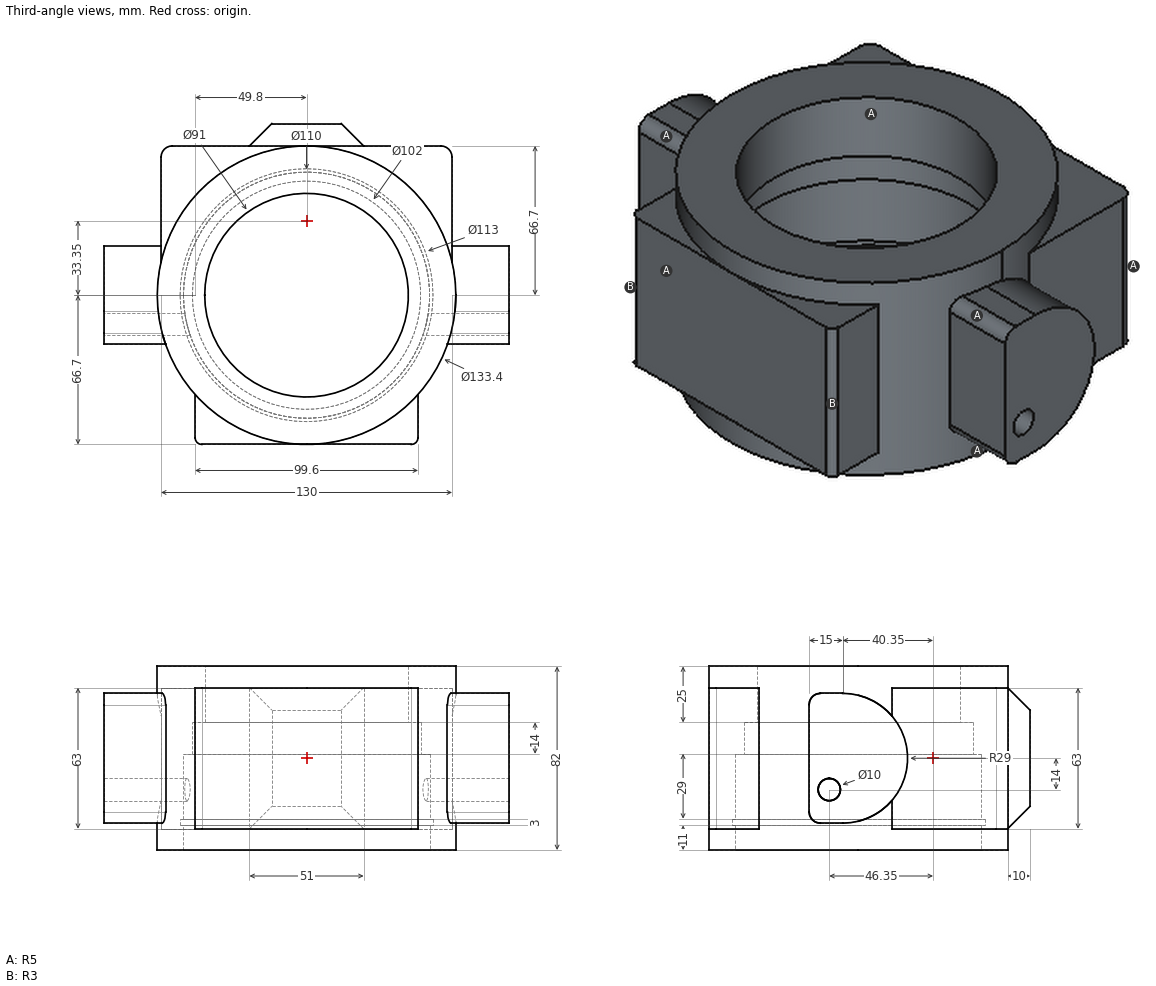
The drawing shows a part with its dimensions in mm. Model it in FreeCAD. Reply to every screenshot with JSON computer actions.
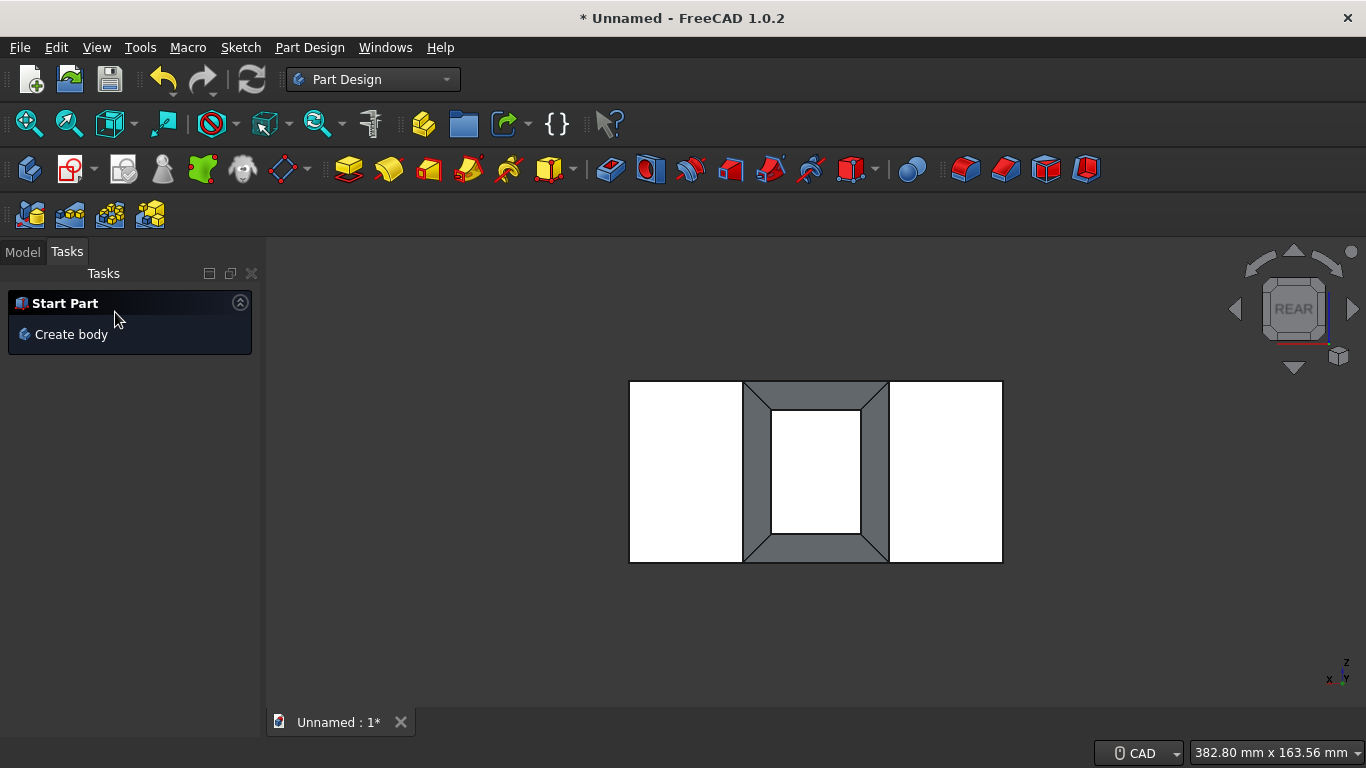
{"action": "left_click", "coordinate": [70, 170]}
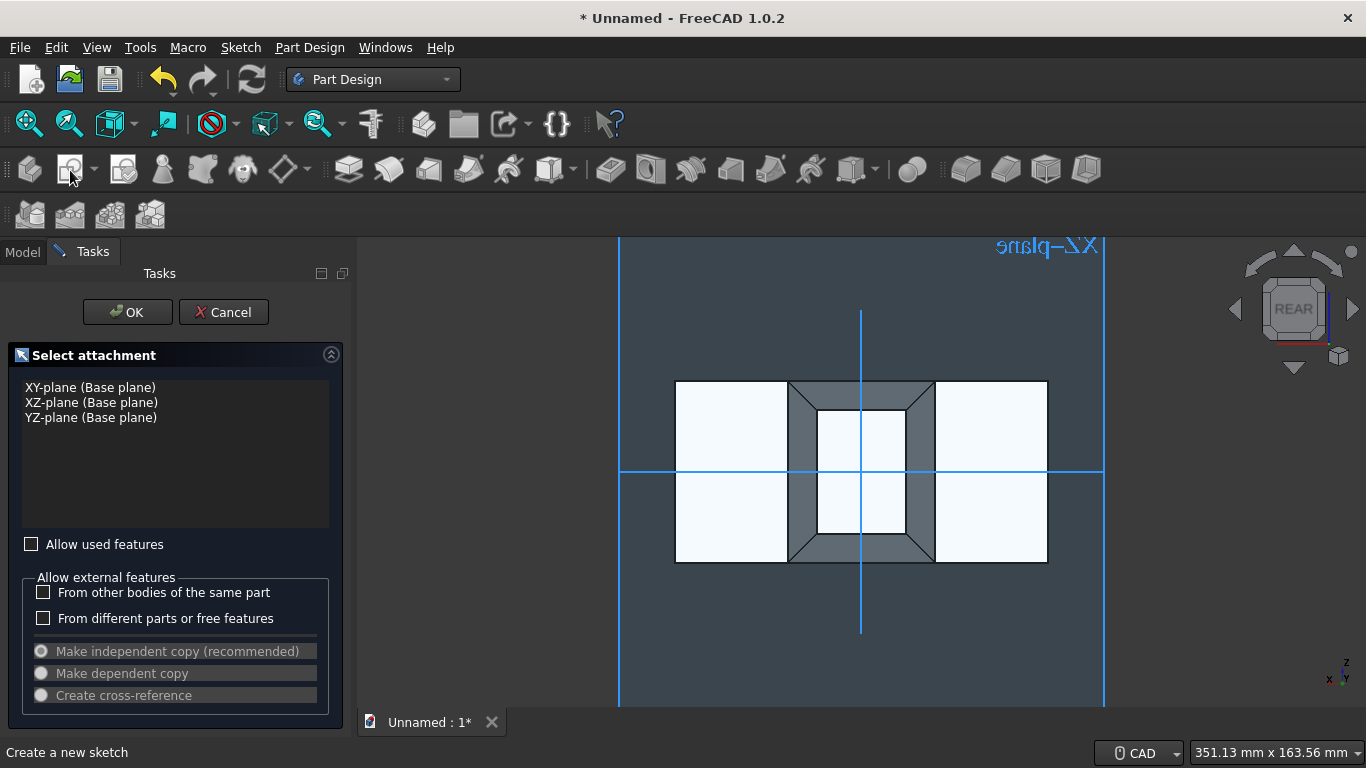
{"action": "left_click", "coordinate": [82, 388]}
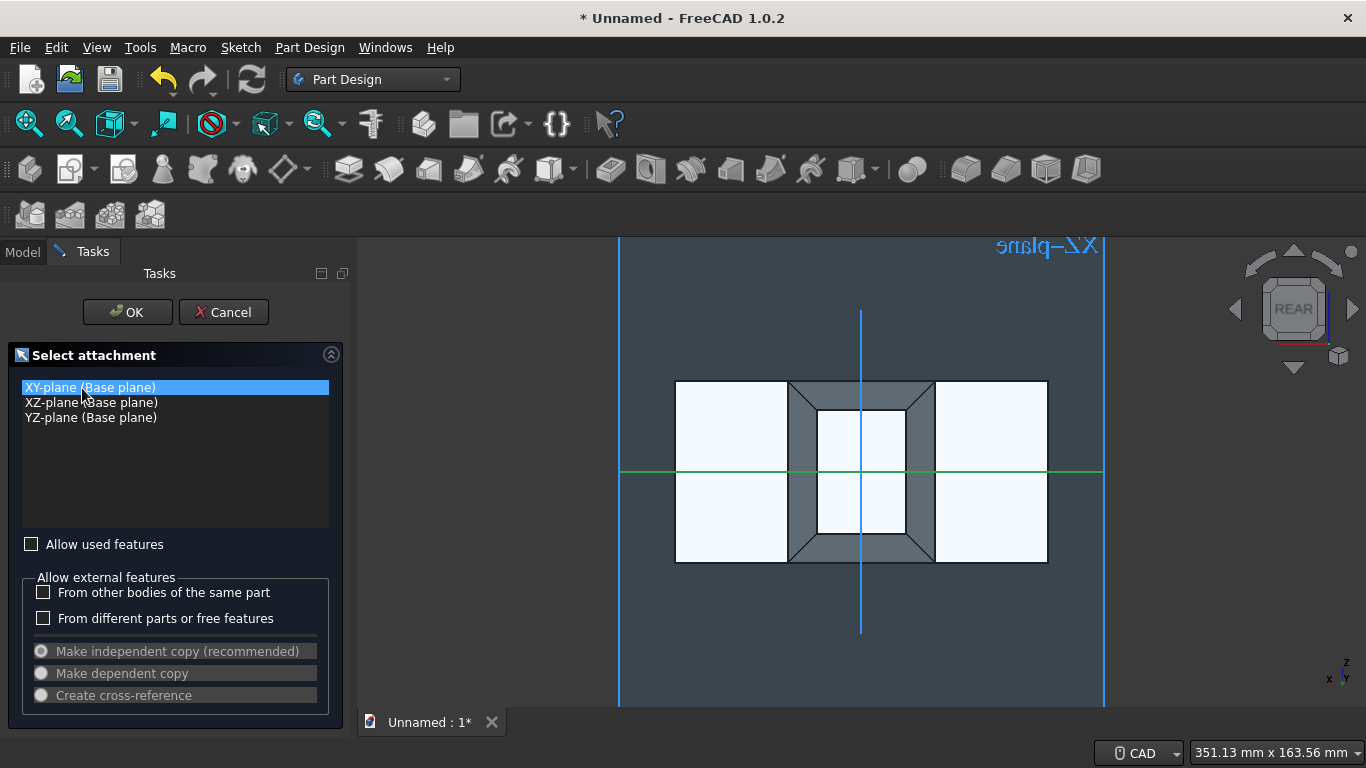
{"action": "left_click", "coordinate": [128, 312]}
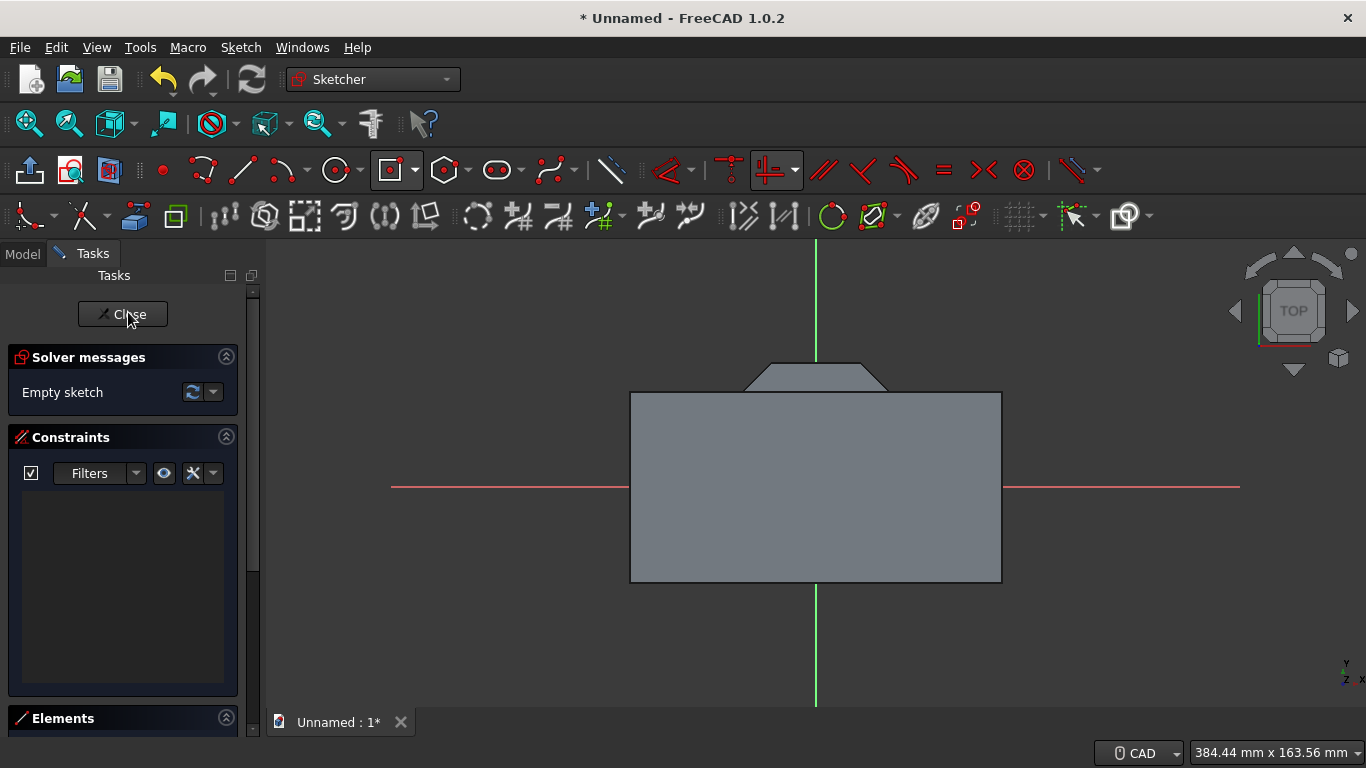
{"action": "key", "text": "q s"}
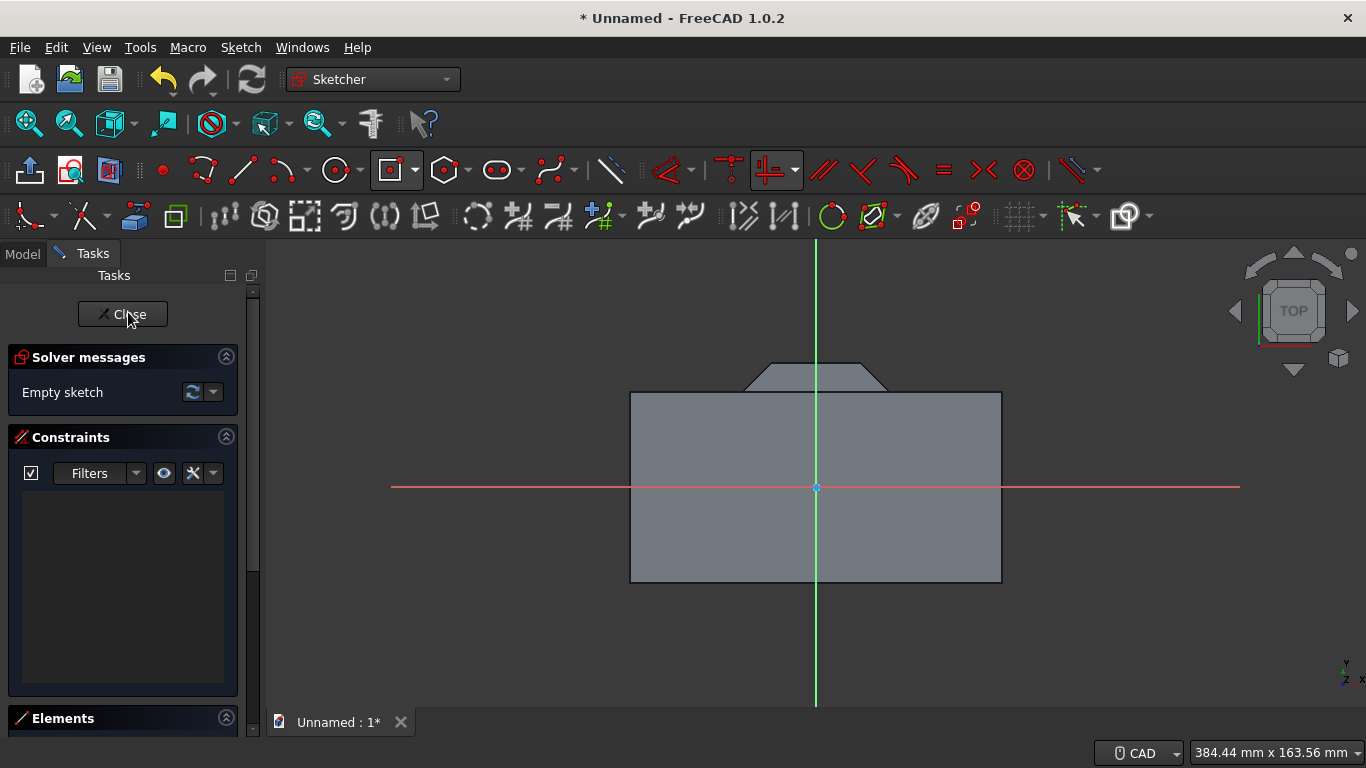
{"action": "scroll", "coordinate": [608, 267], "scroll_direction": "down", "scroll_amount": 2}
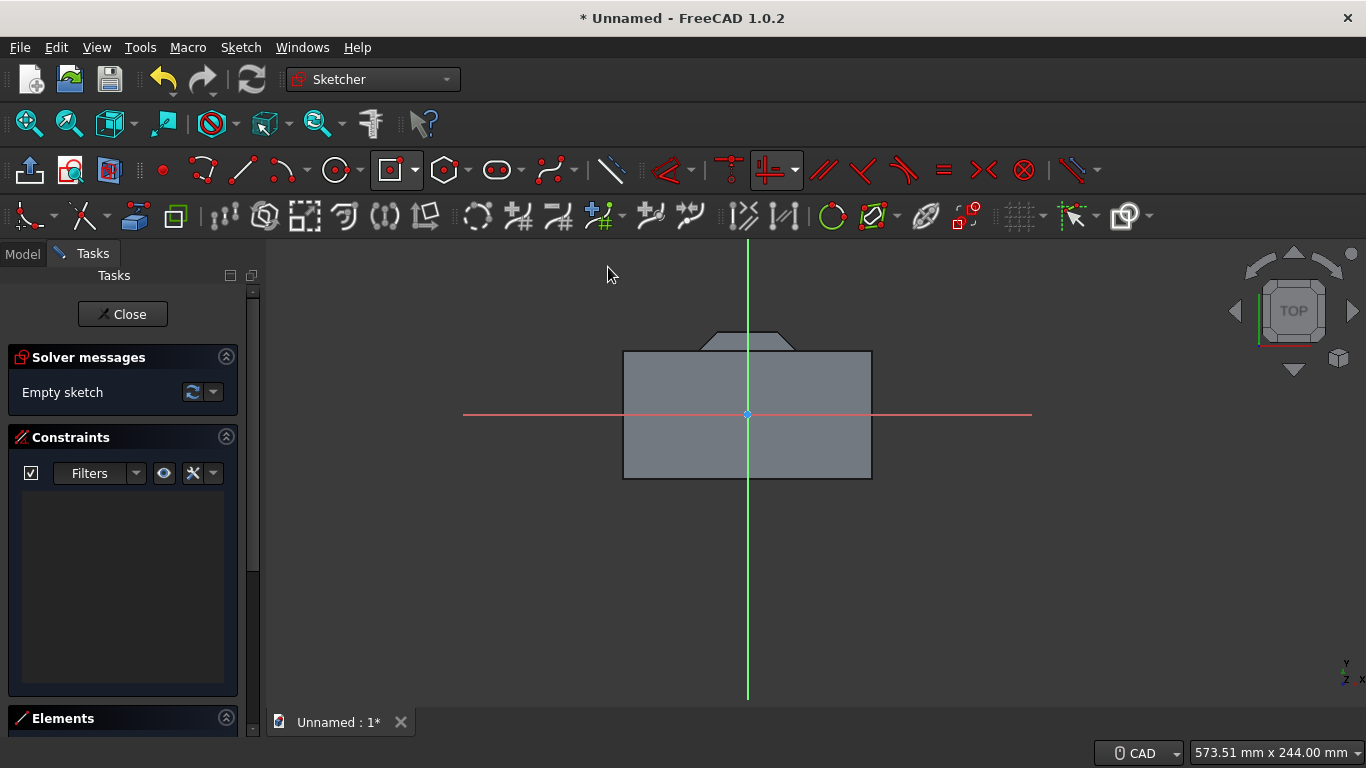
{"action": "scroll", "coordinate": [748, 587], "scroll_direction": "up", "scroll_amount": 2}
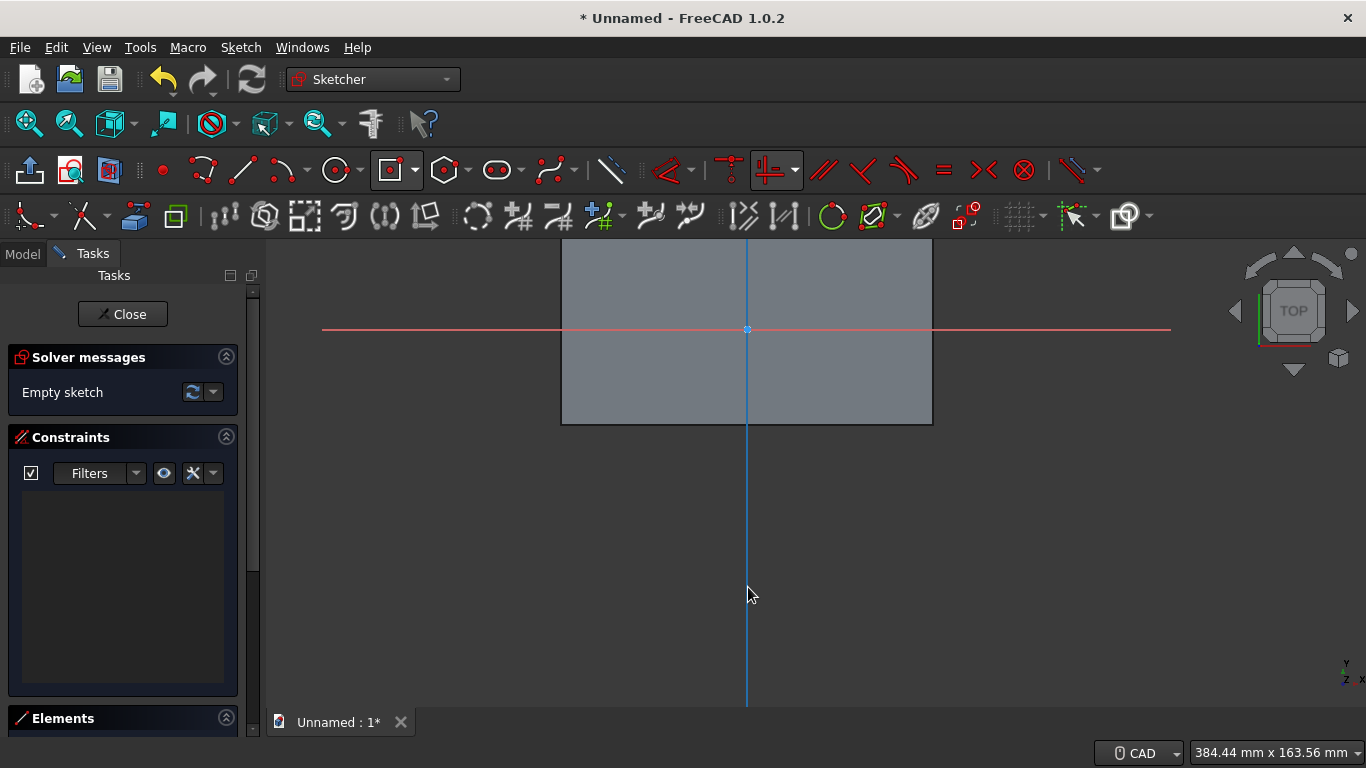
{"action": "key", "text": "g r"}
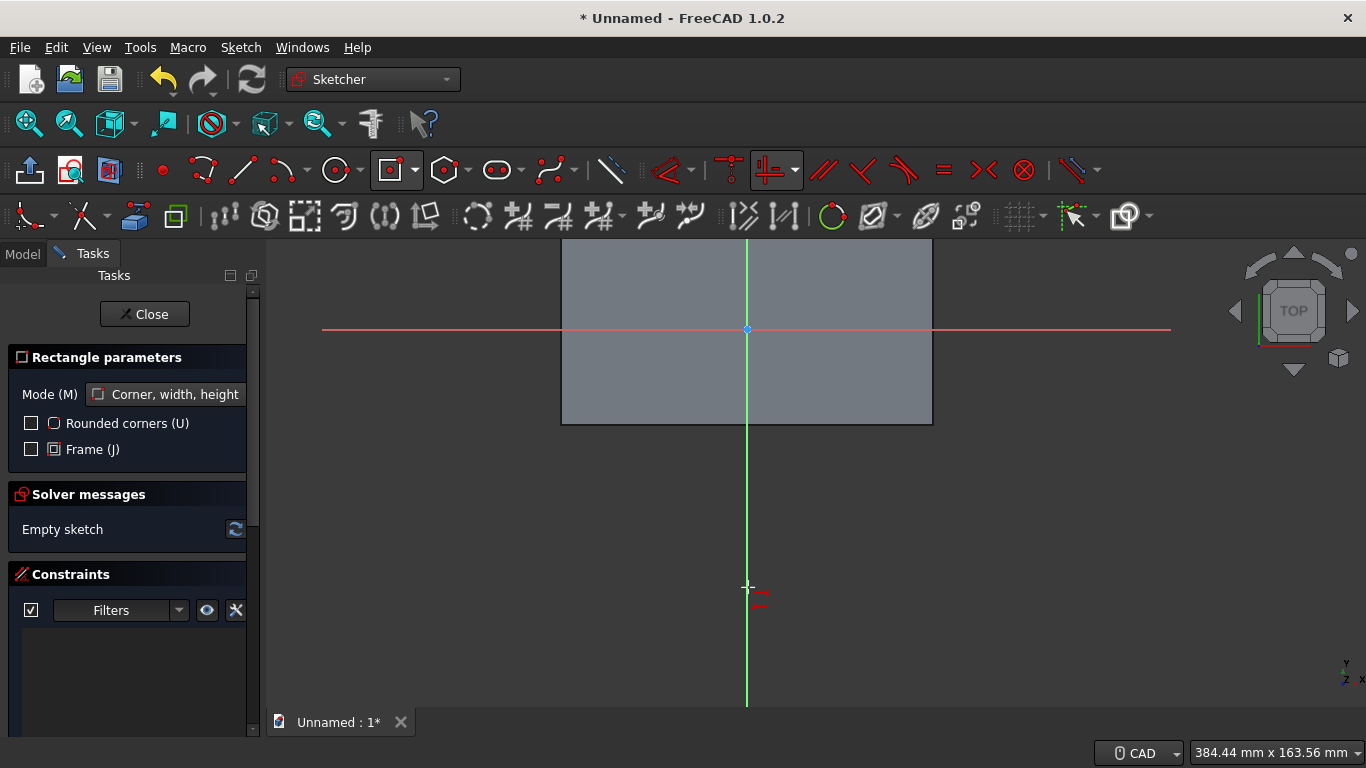
{"action": "left_click", "coordinate": [605, 425]}
{"action": "left_click", "coordinate": [890, 616]}
{"action": "key", "text": "Escape"}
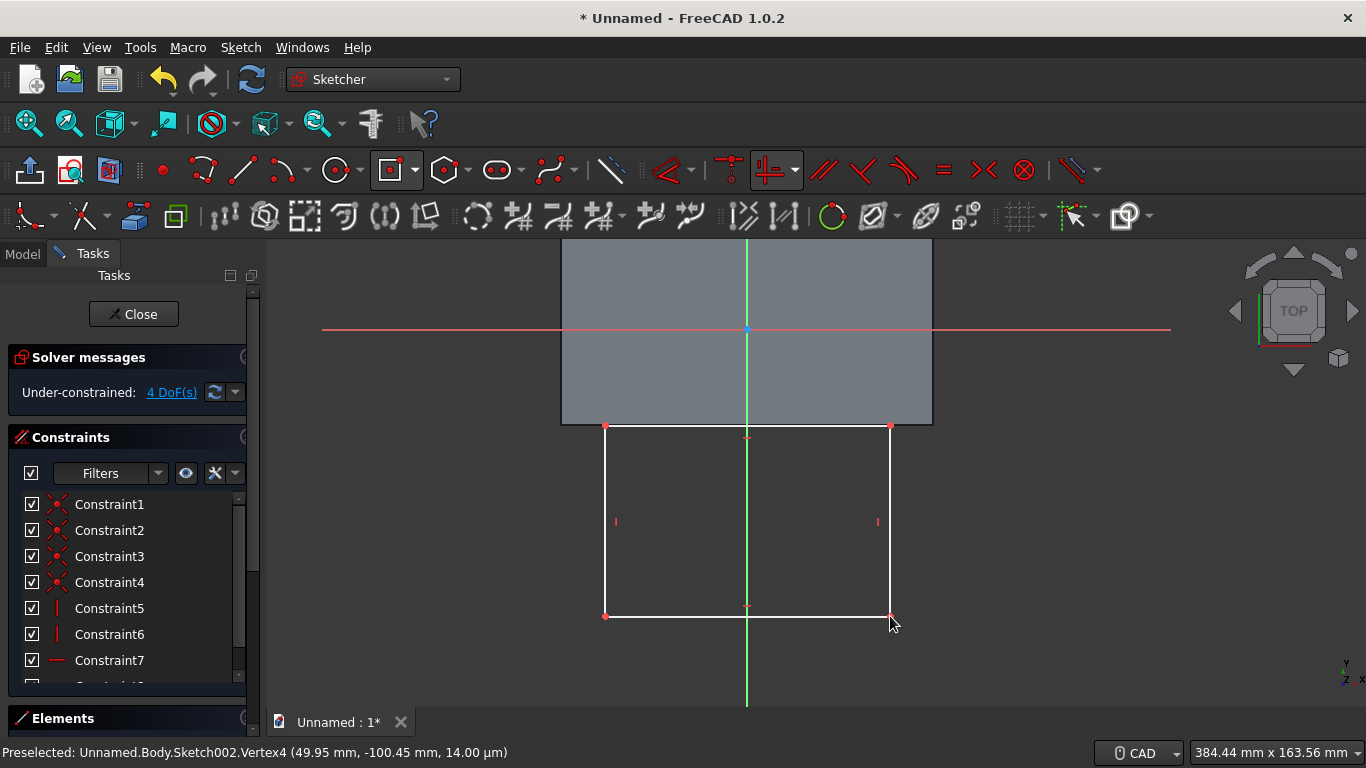
{"action": "key", "text": "d"}